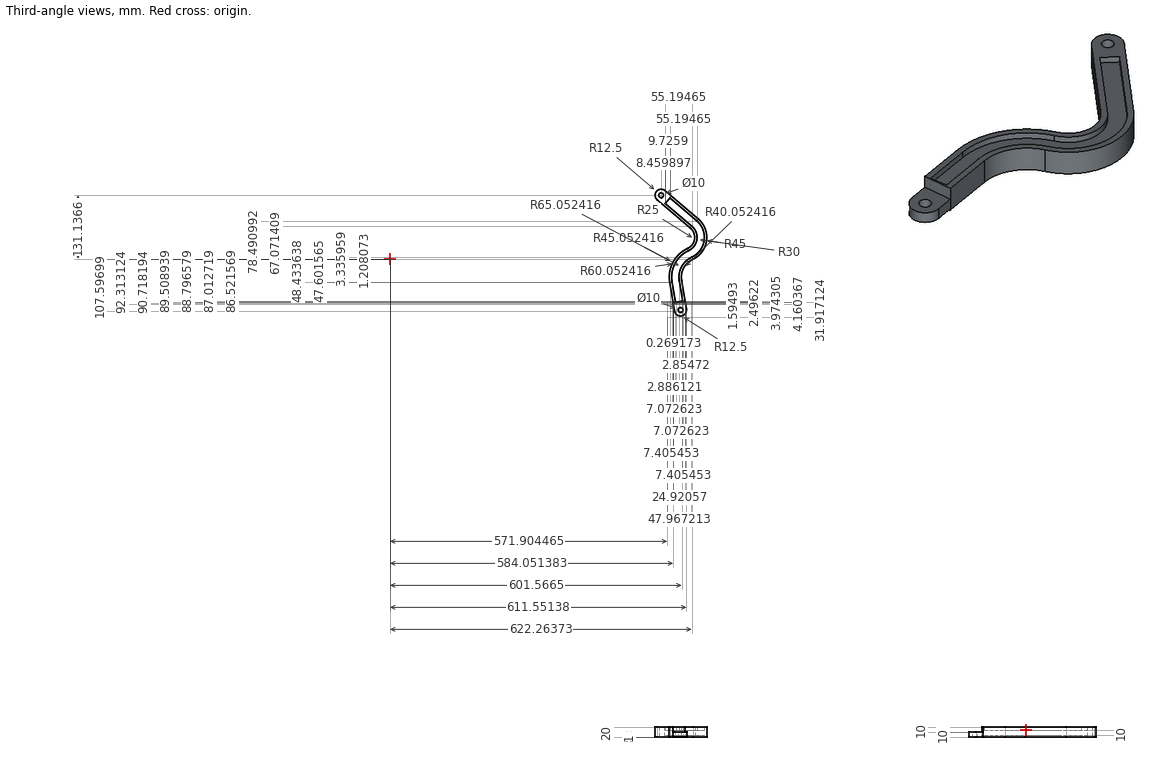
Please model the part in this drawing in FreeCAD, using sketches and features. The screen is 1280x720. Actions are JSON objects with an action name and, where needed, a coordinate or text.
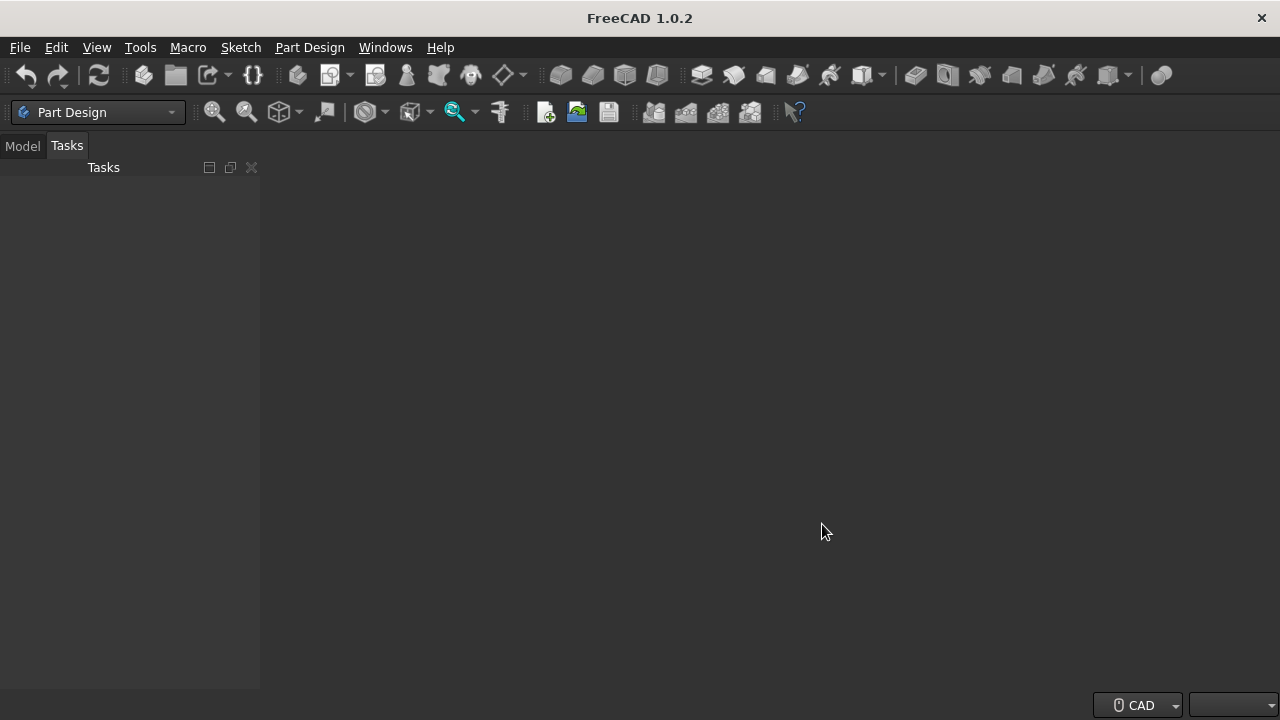
{"action": "left_click", "coordinate": [546, 112]}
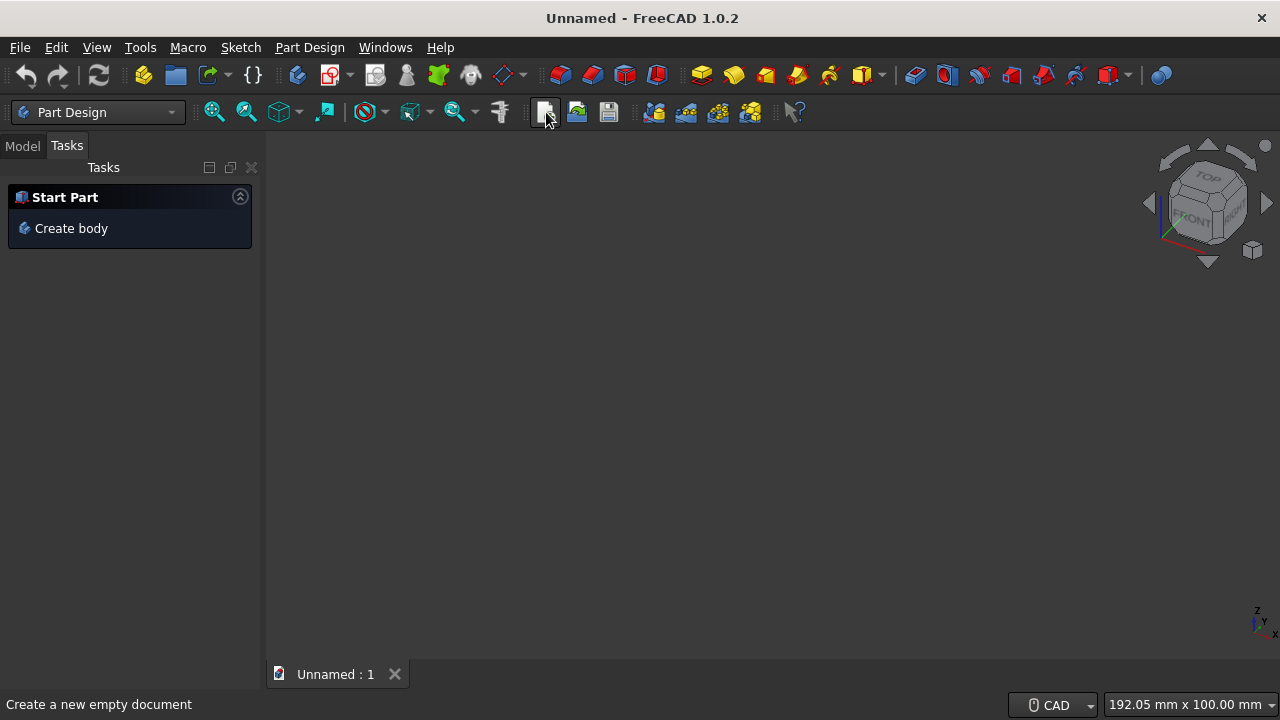
{"action": "left_click", "coordinate": [330, 76]}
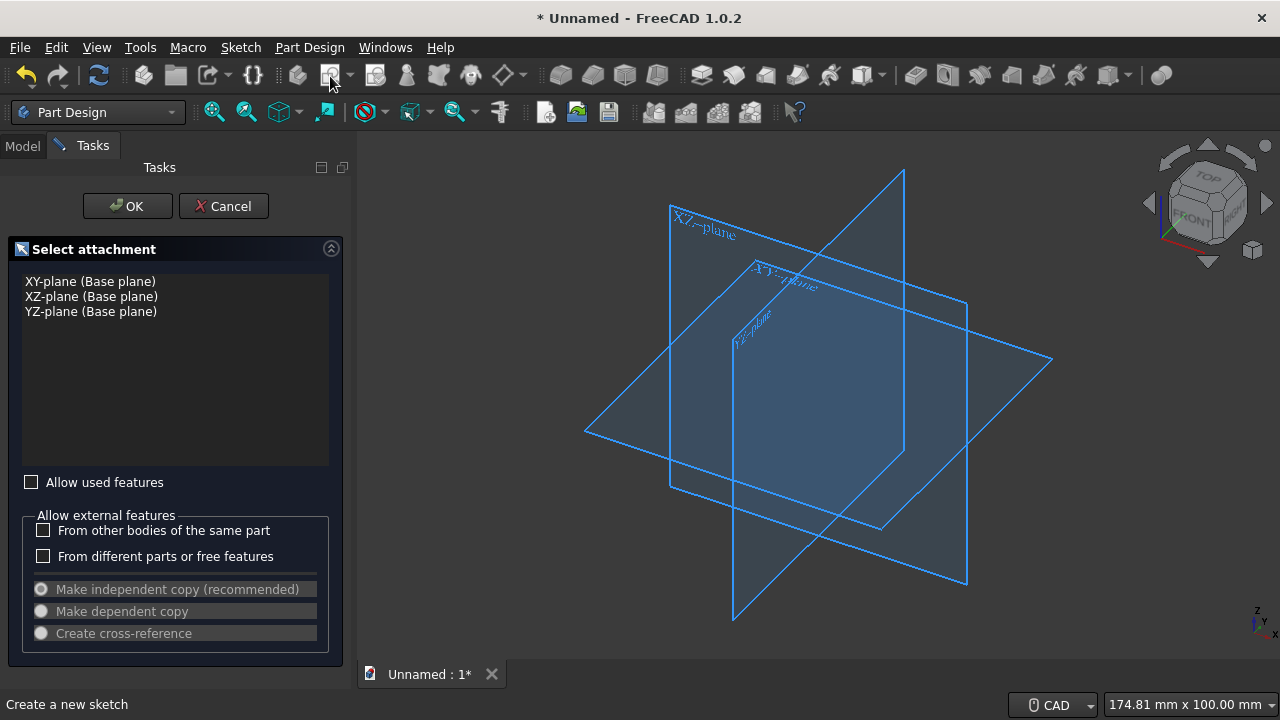
{"action": "left_click", "coordinate": [82, 282]}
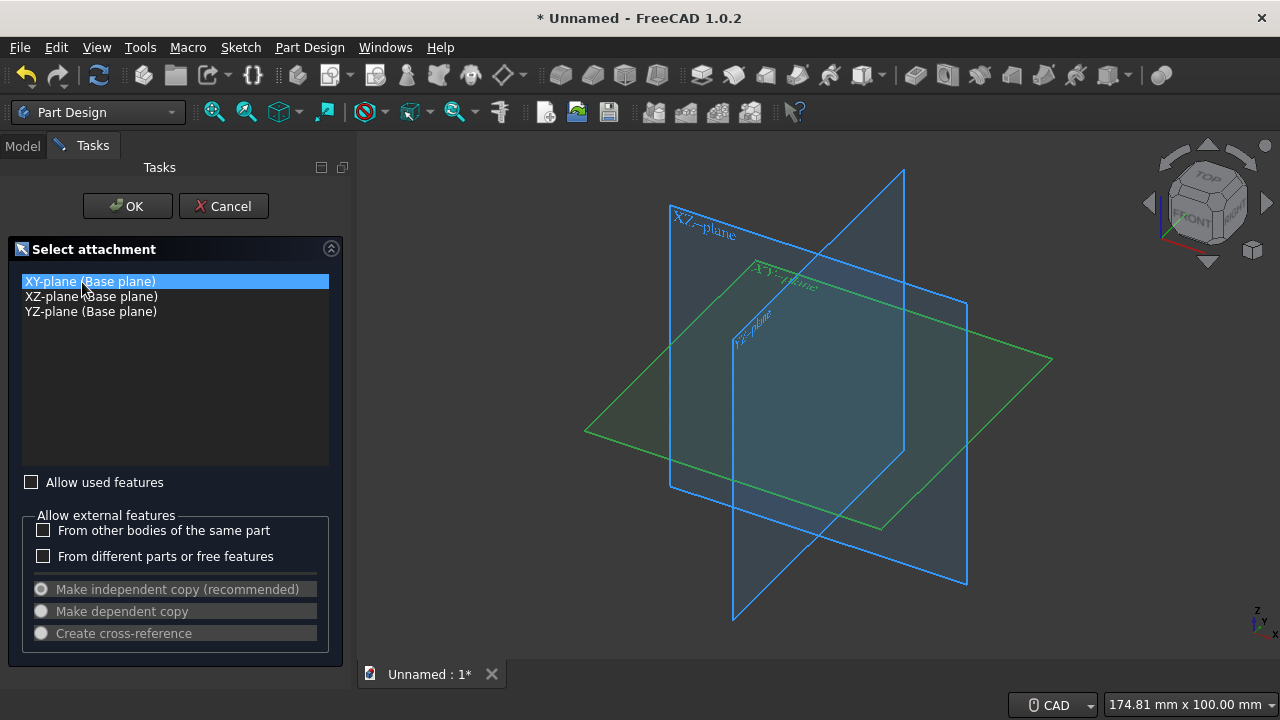
{"action": "left_click", "coordinate": [128, 206]}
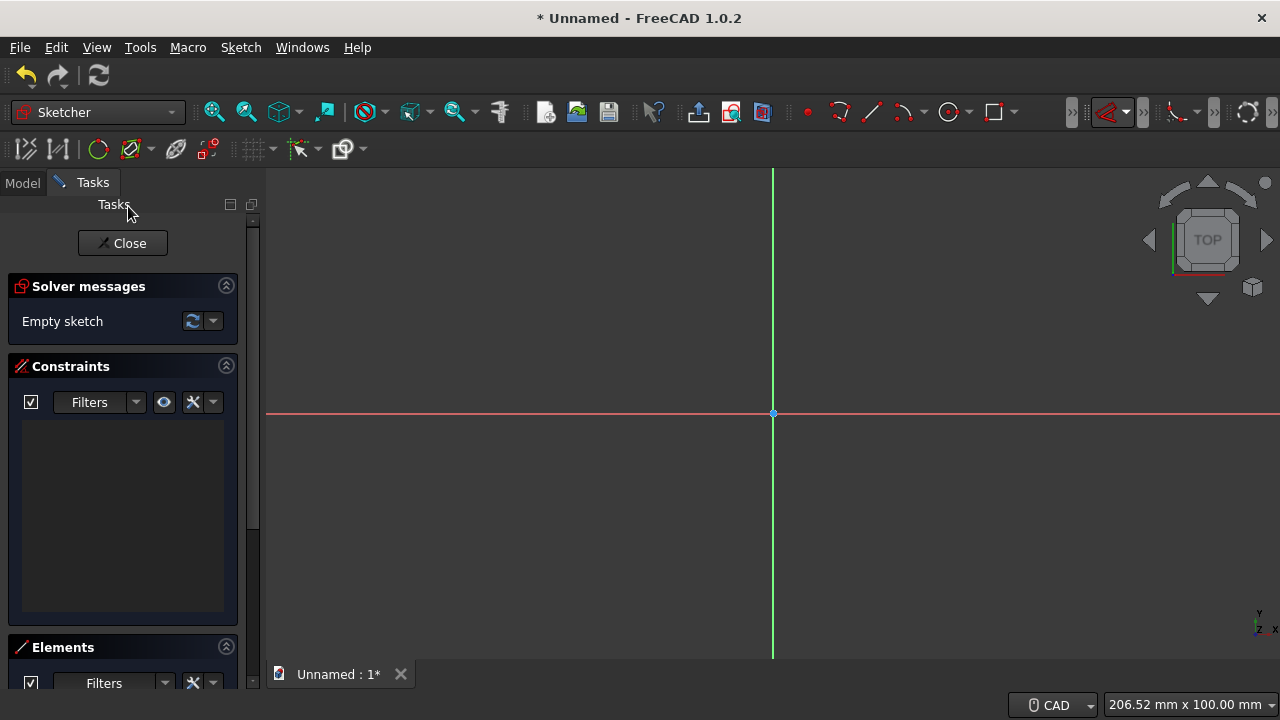
{"action": "scroll", "coordinate": [294, 436], "scroll_direction": "down", "scroll_amount": 8}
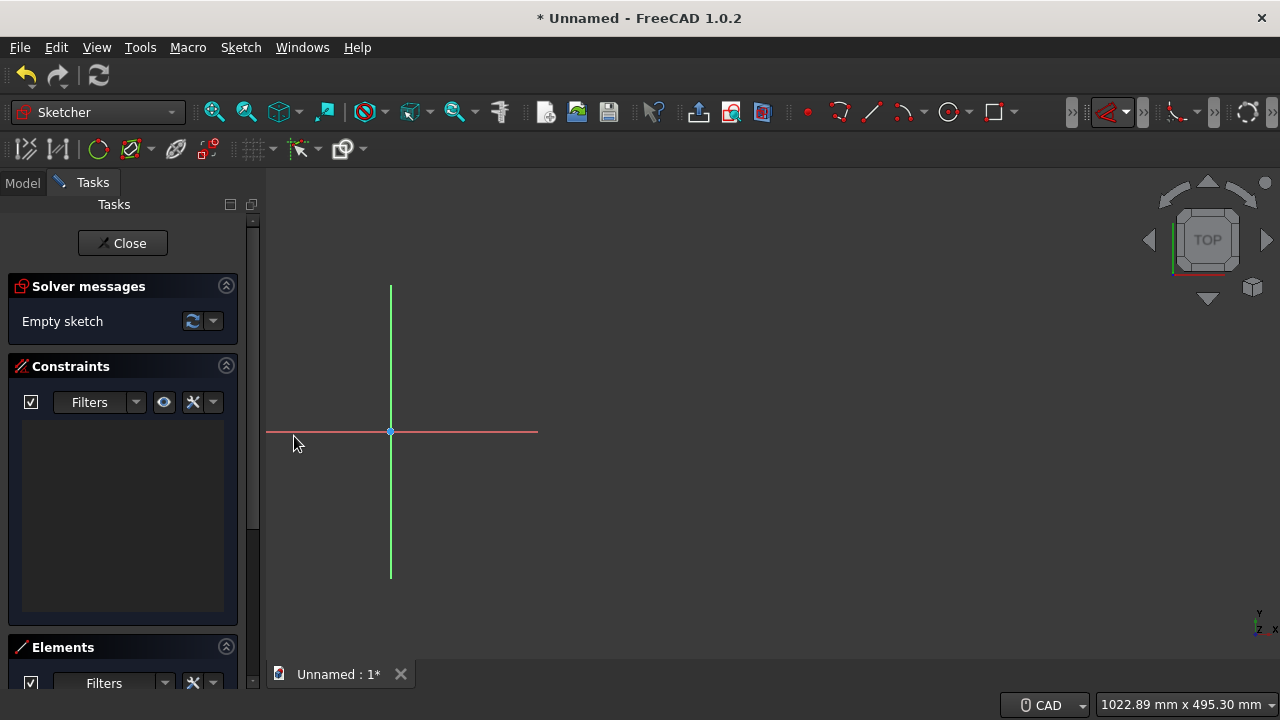
{"action": "scroll", "coordinate": [1115, 415], "scroll_direction": "up", "scroll_amount": 2}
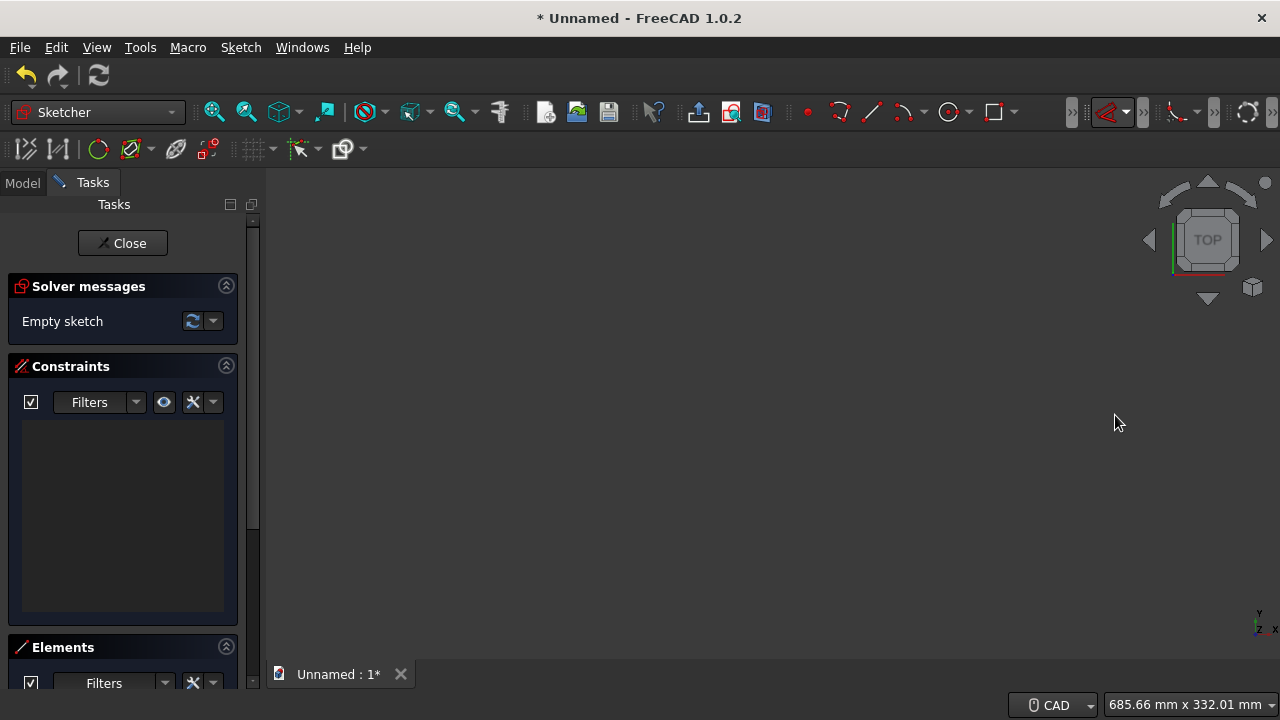
{"action": "left_click", "coordinate": [840, 112]}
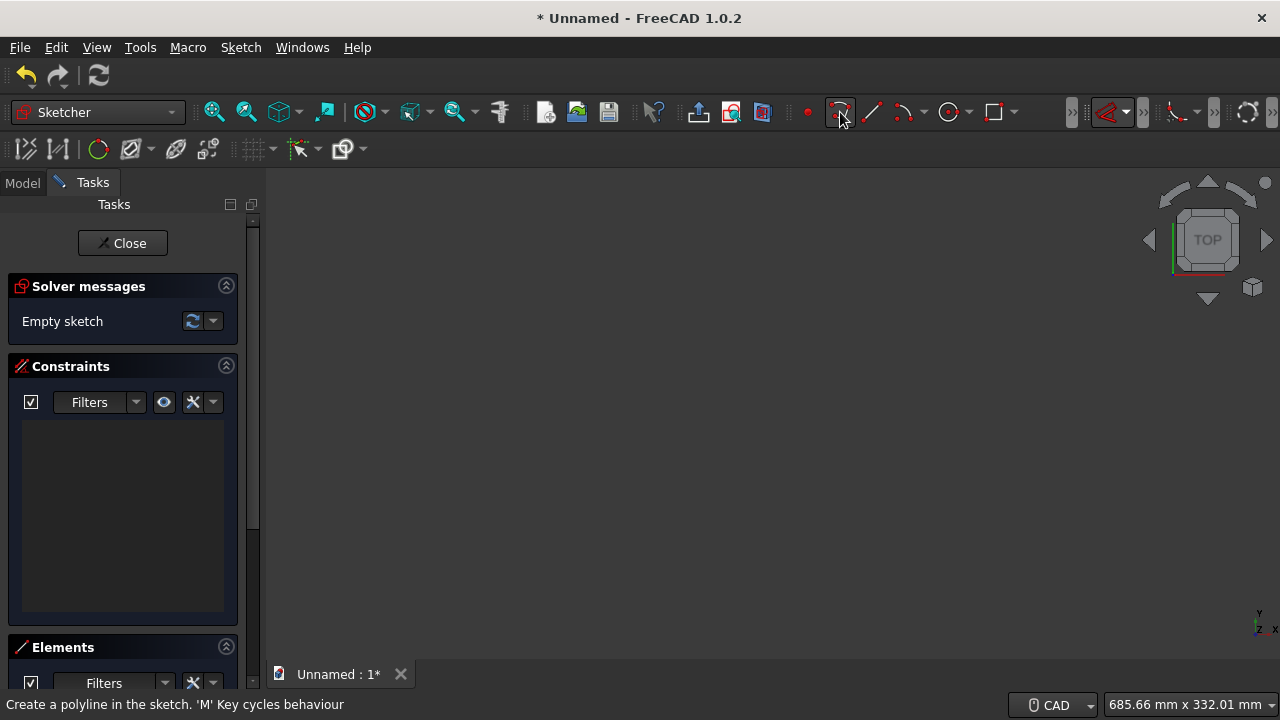
{"action": "left_click", "coordinate": [895, 510]}
{"action": "left_click", "coordinate": [905, 572]}
{"action": "left_click", "coordinate": [927, 569]}
{"action": "left_click", "coordinate": [916, 507]}
{"action": "right_click", "coordinate": [916, 507]}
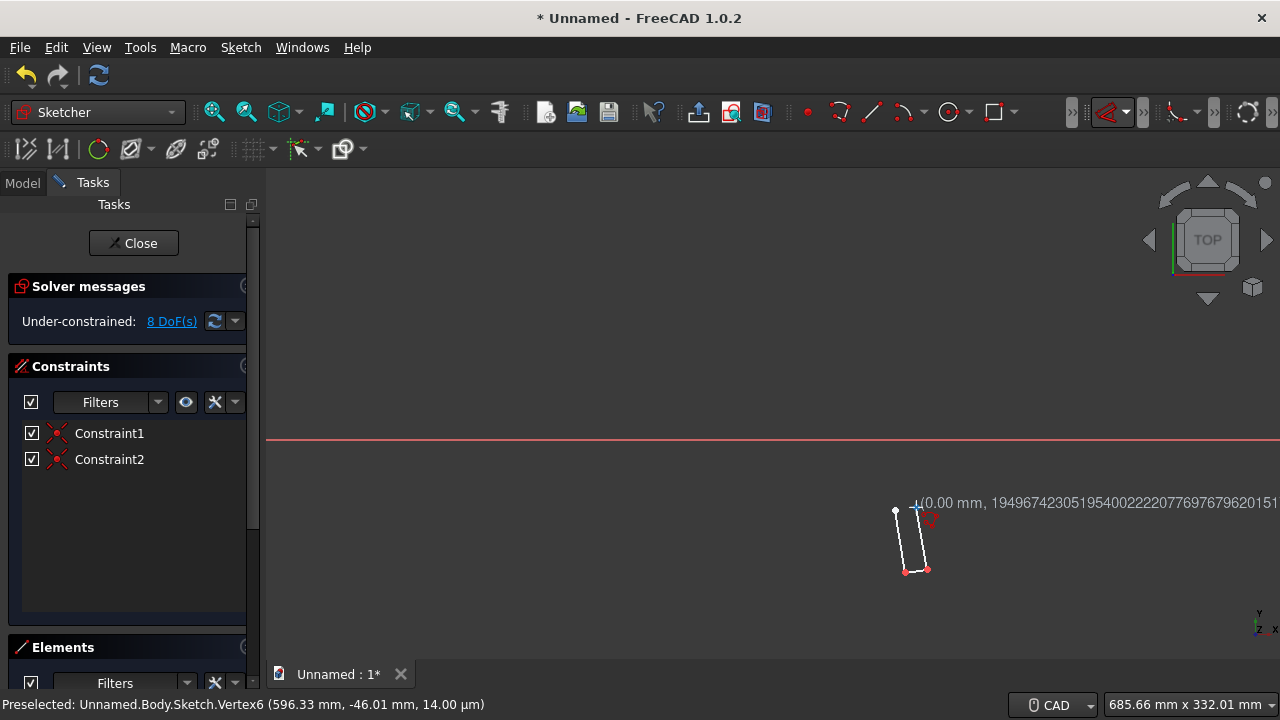
{"action": "left_click", "coordinate": [970, 324]}
{"action": "left_click", "coordinate": [888, 254]}
{"action": "left_click", "coordinate": [874, 271]}
{"action": "left_click", "coordinate": [955, 341]}
{"action": "right_click", "coordinate": [955, 341]}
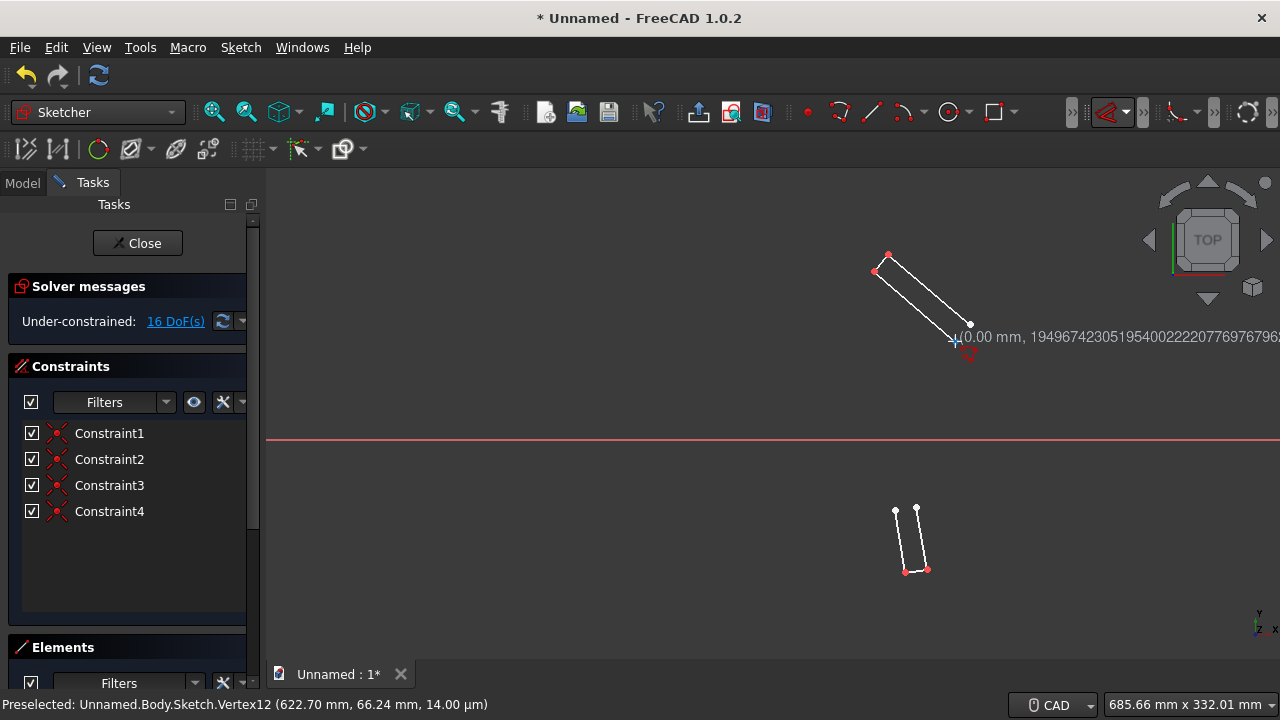
{"action": "key", "text": "g 3 a"}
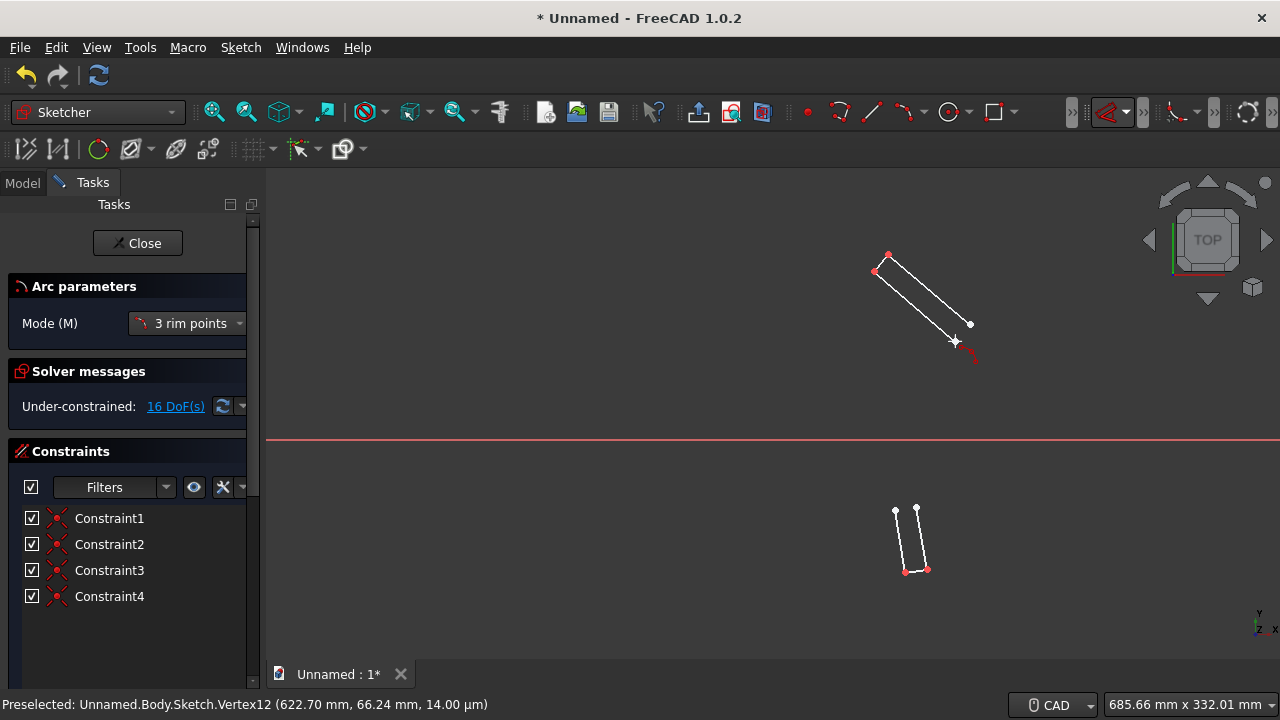
{"action": "left_click", "coordinate": [916, 508]}